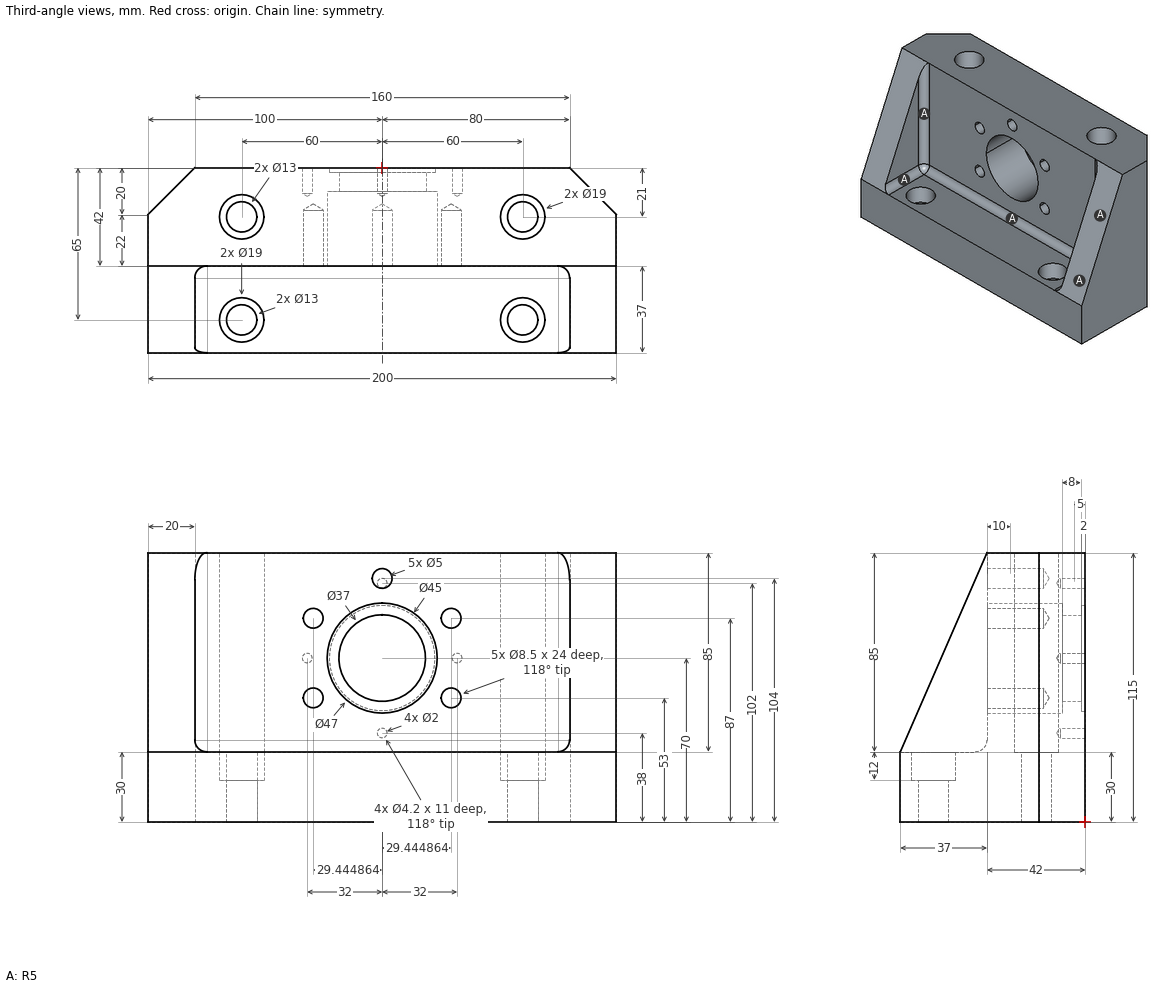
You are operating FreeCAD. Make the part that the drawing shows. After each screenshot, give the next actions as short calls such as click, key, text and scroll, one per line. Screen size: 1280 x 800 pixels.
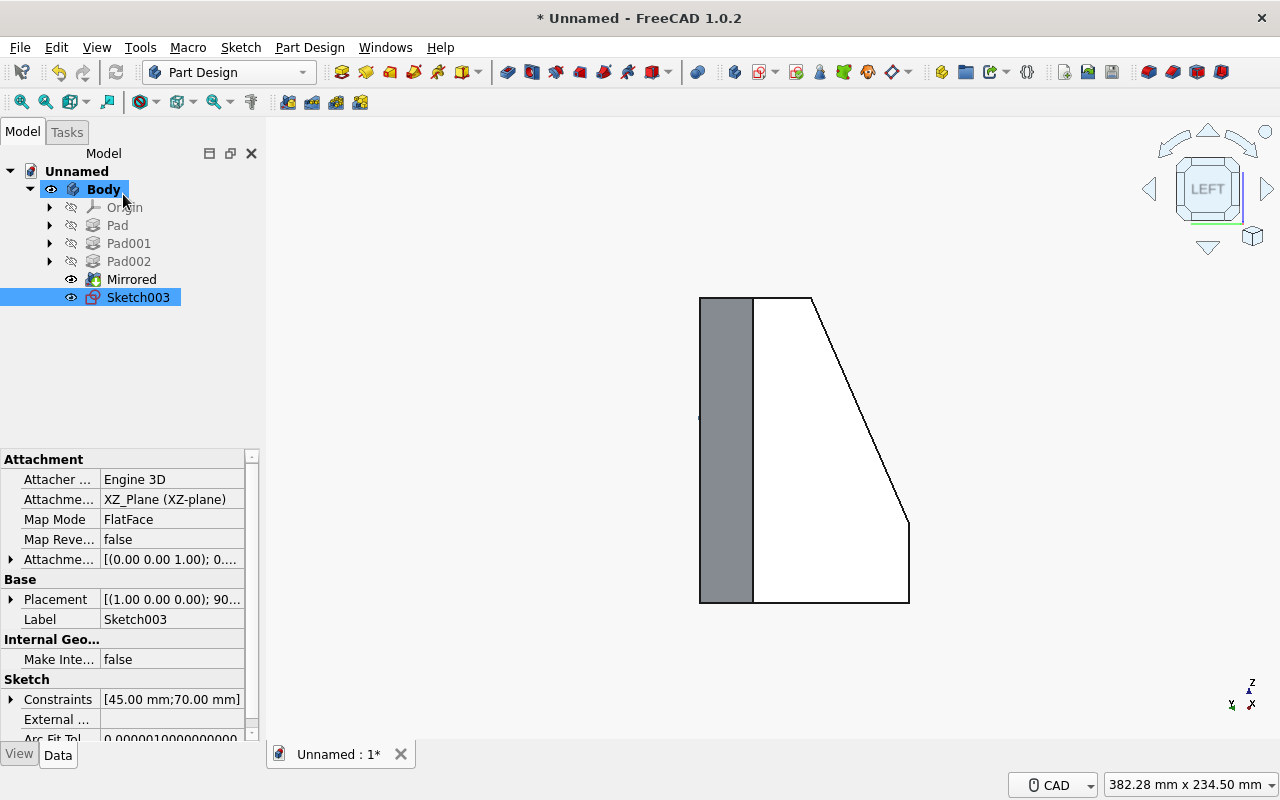
click(508, 72)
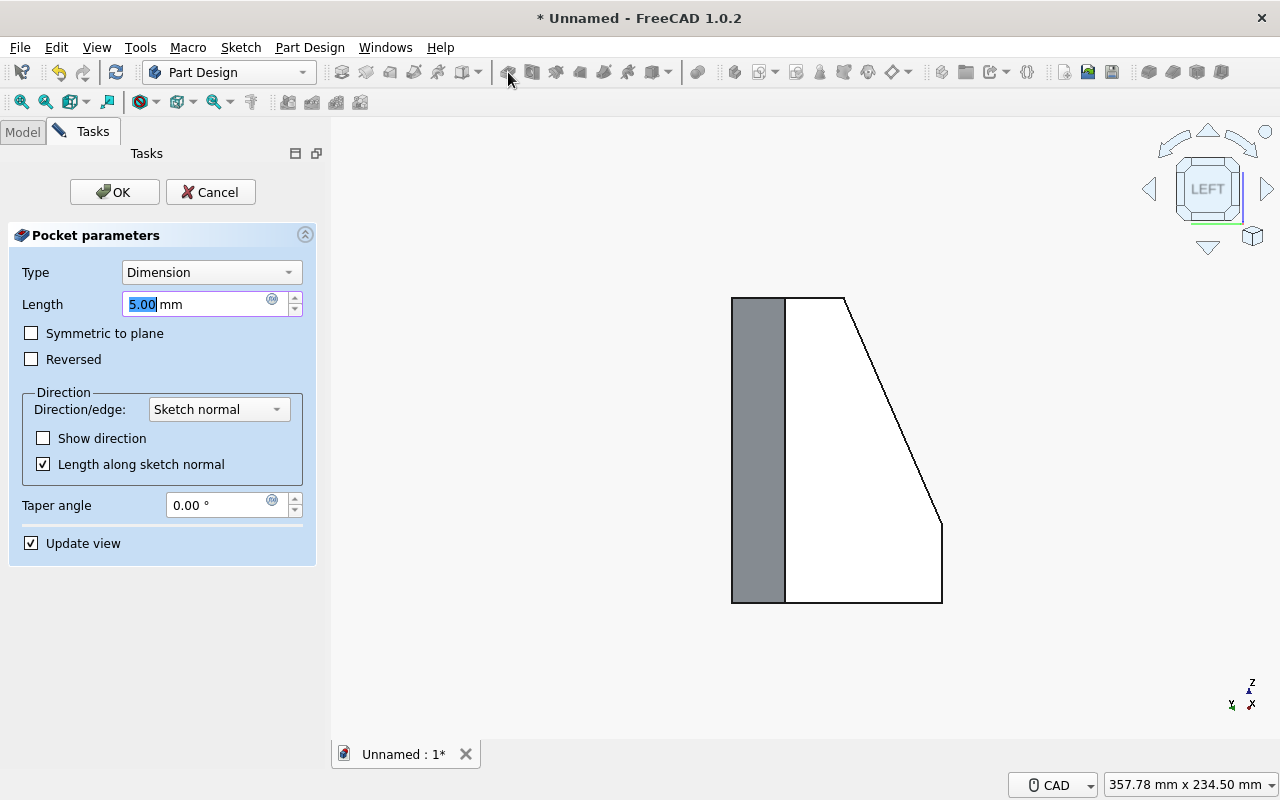
text(2)
key(Tab)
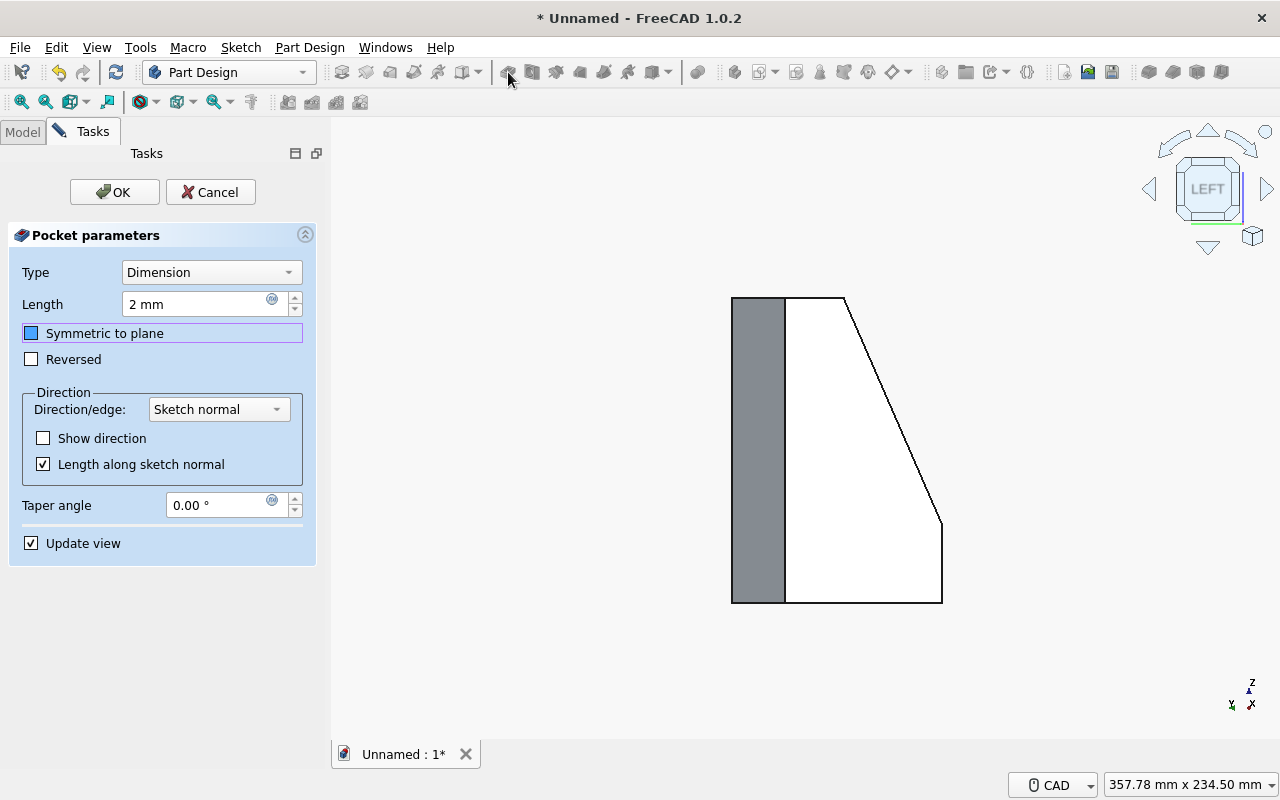
click(30, 359)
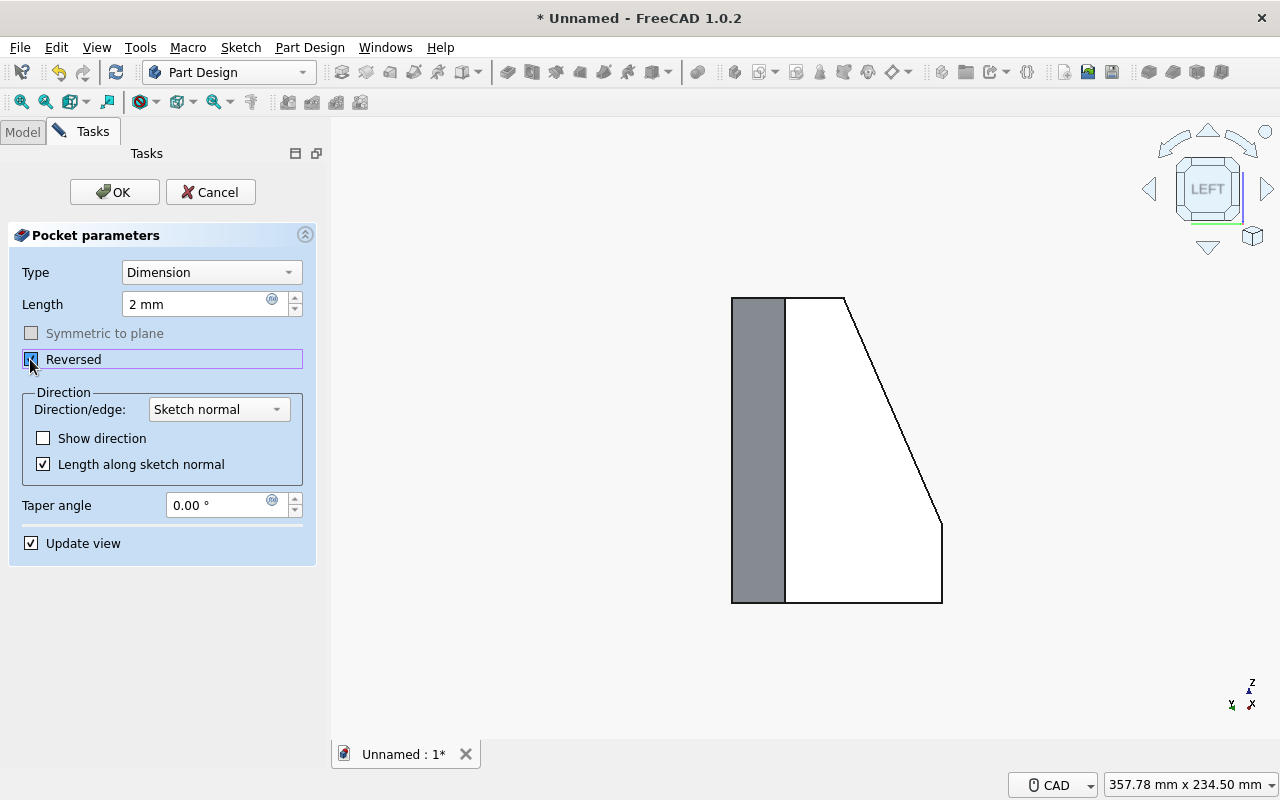
click(115, 192)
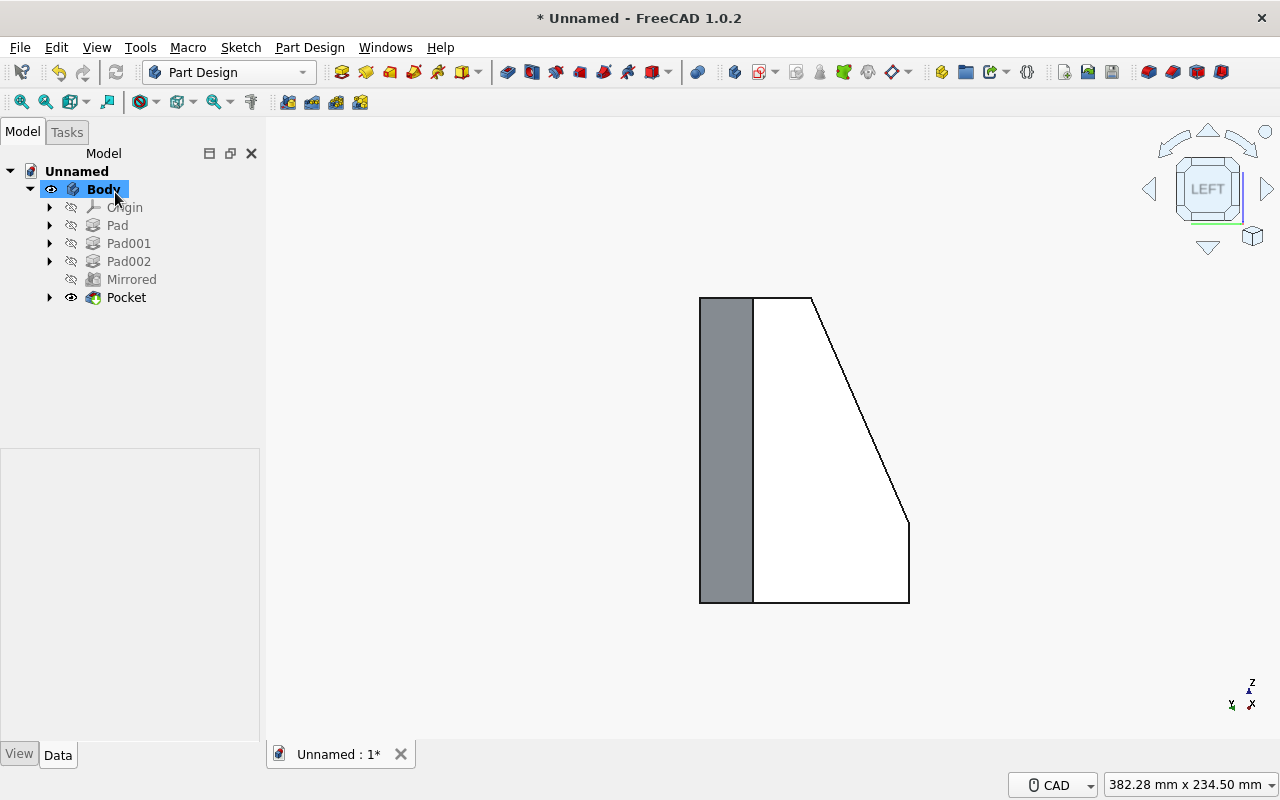
key(4)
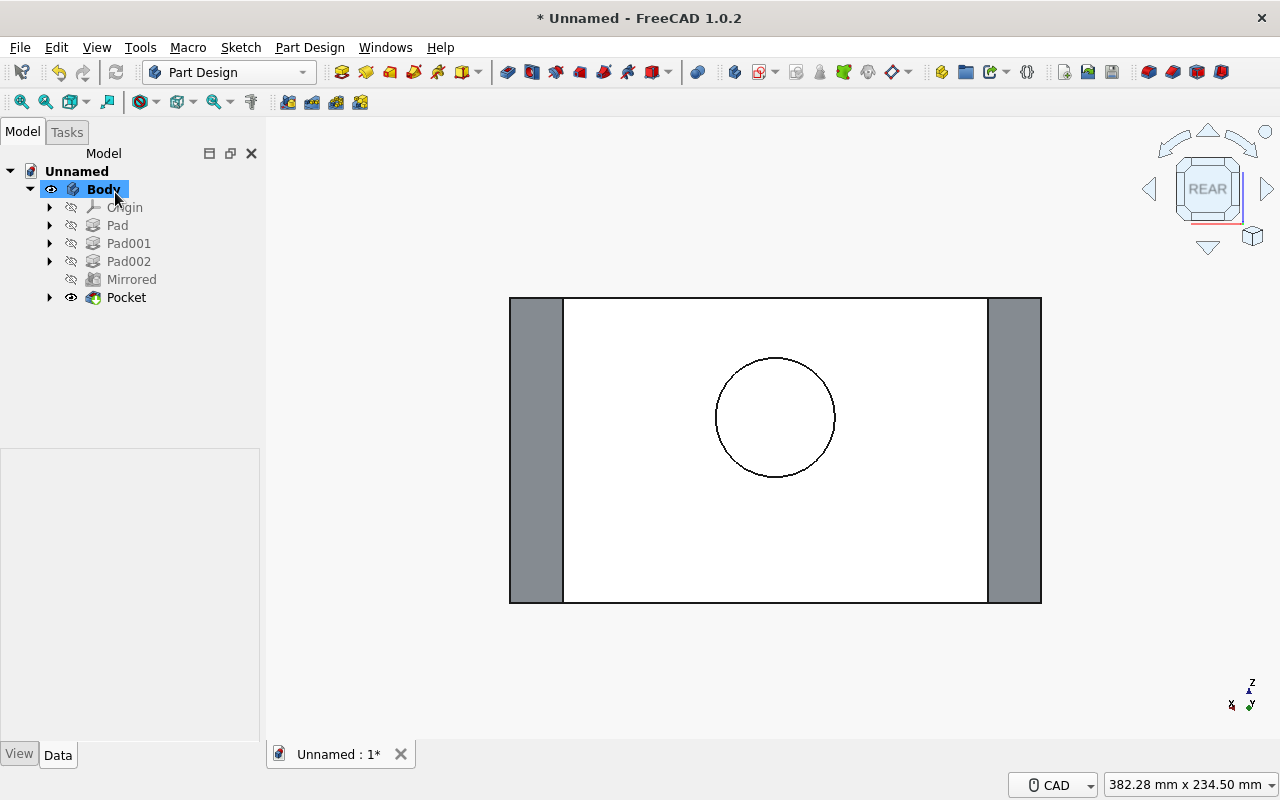
click(775, 417)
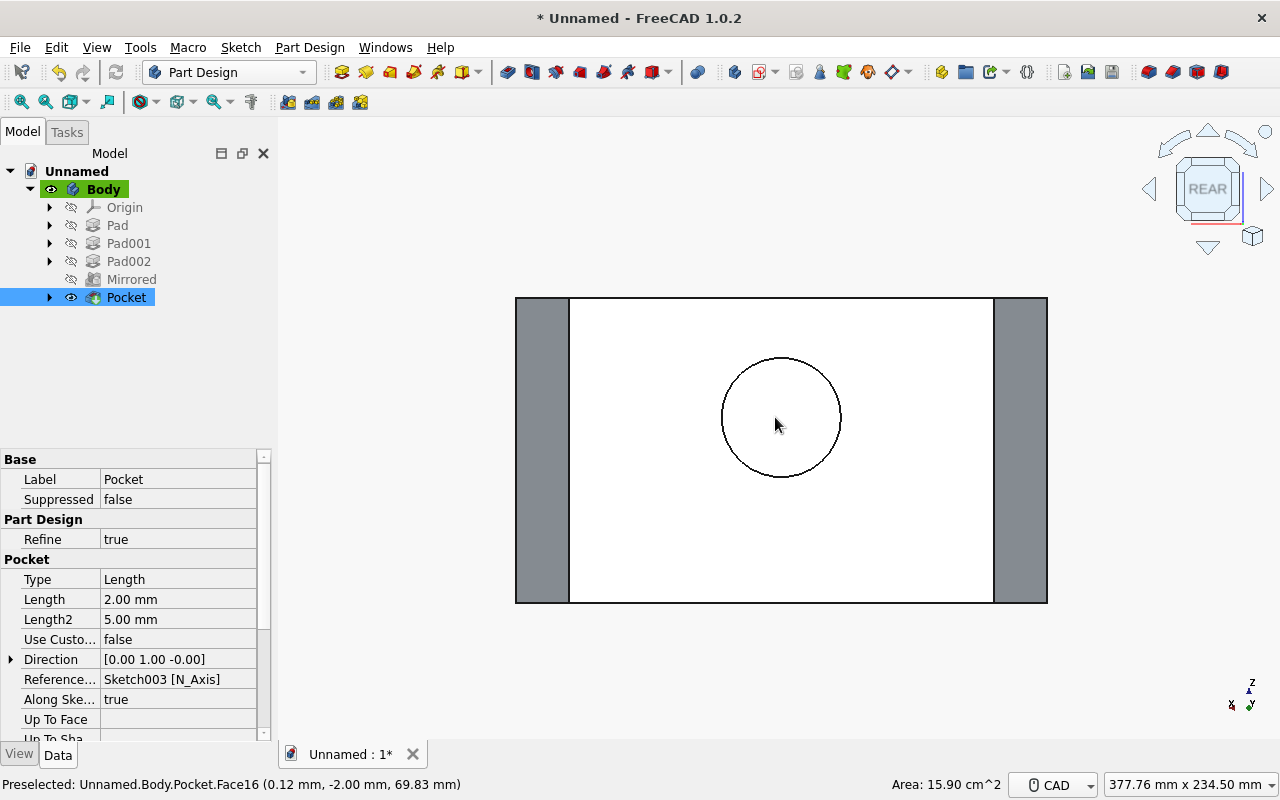
click(760, 72)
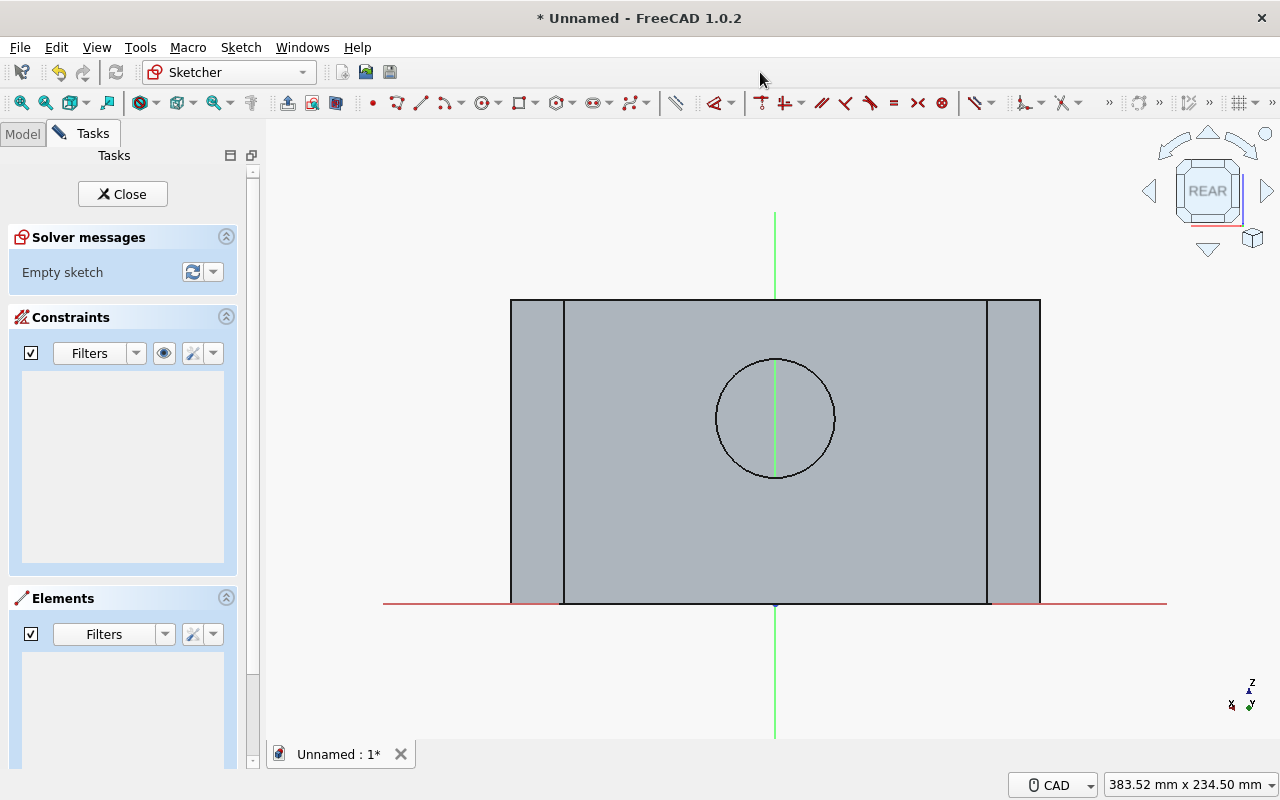
scroll(861, 557, up, 3)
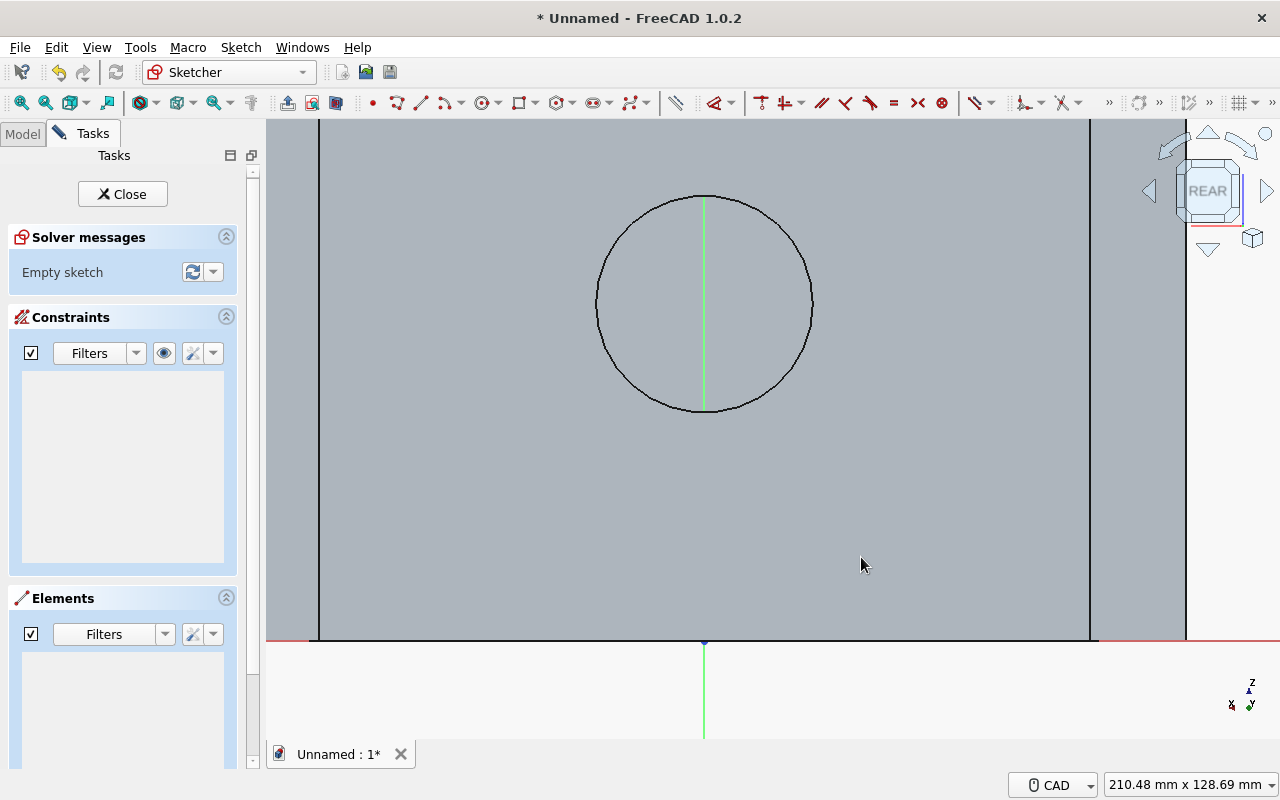
click(482, 104)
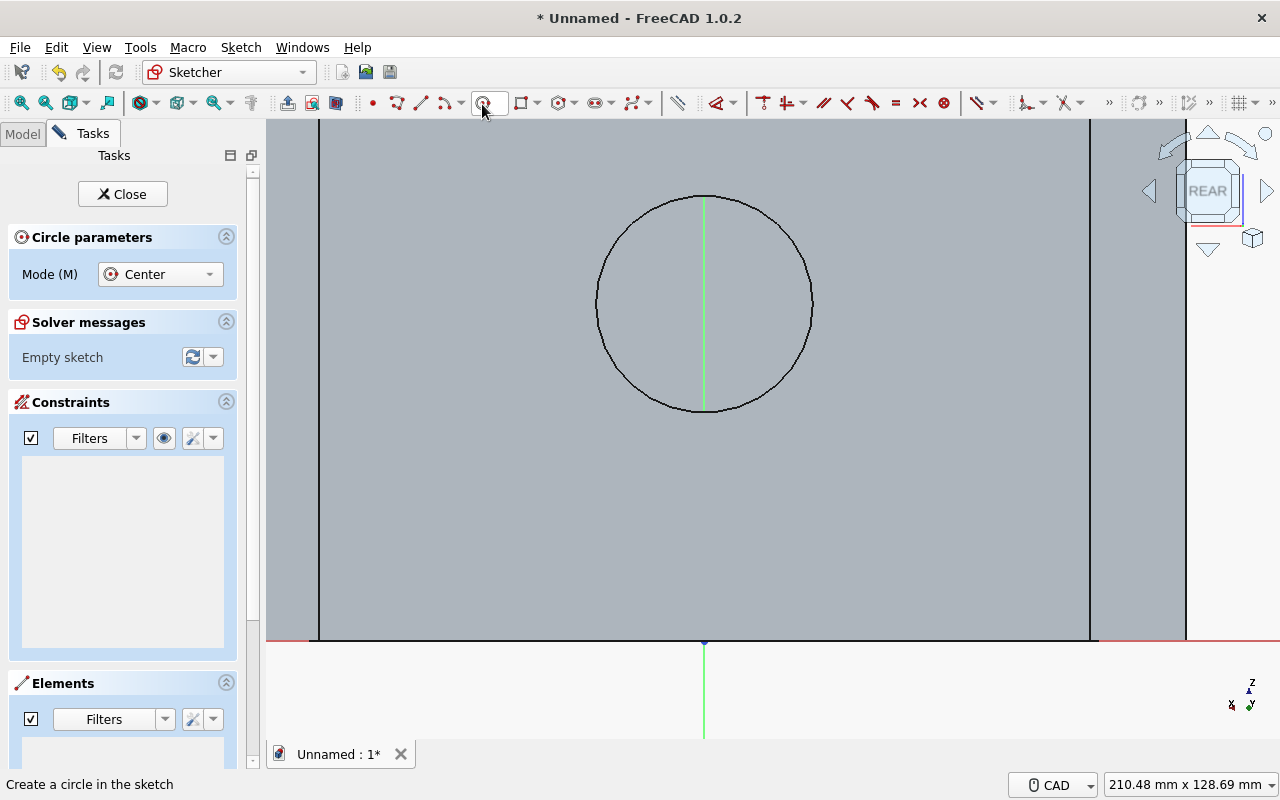
click(704, 304)
move(767, 241)